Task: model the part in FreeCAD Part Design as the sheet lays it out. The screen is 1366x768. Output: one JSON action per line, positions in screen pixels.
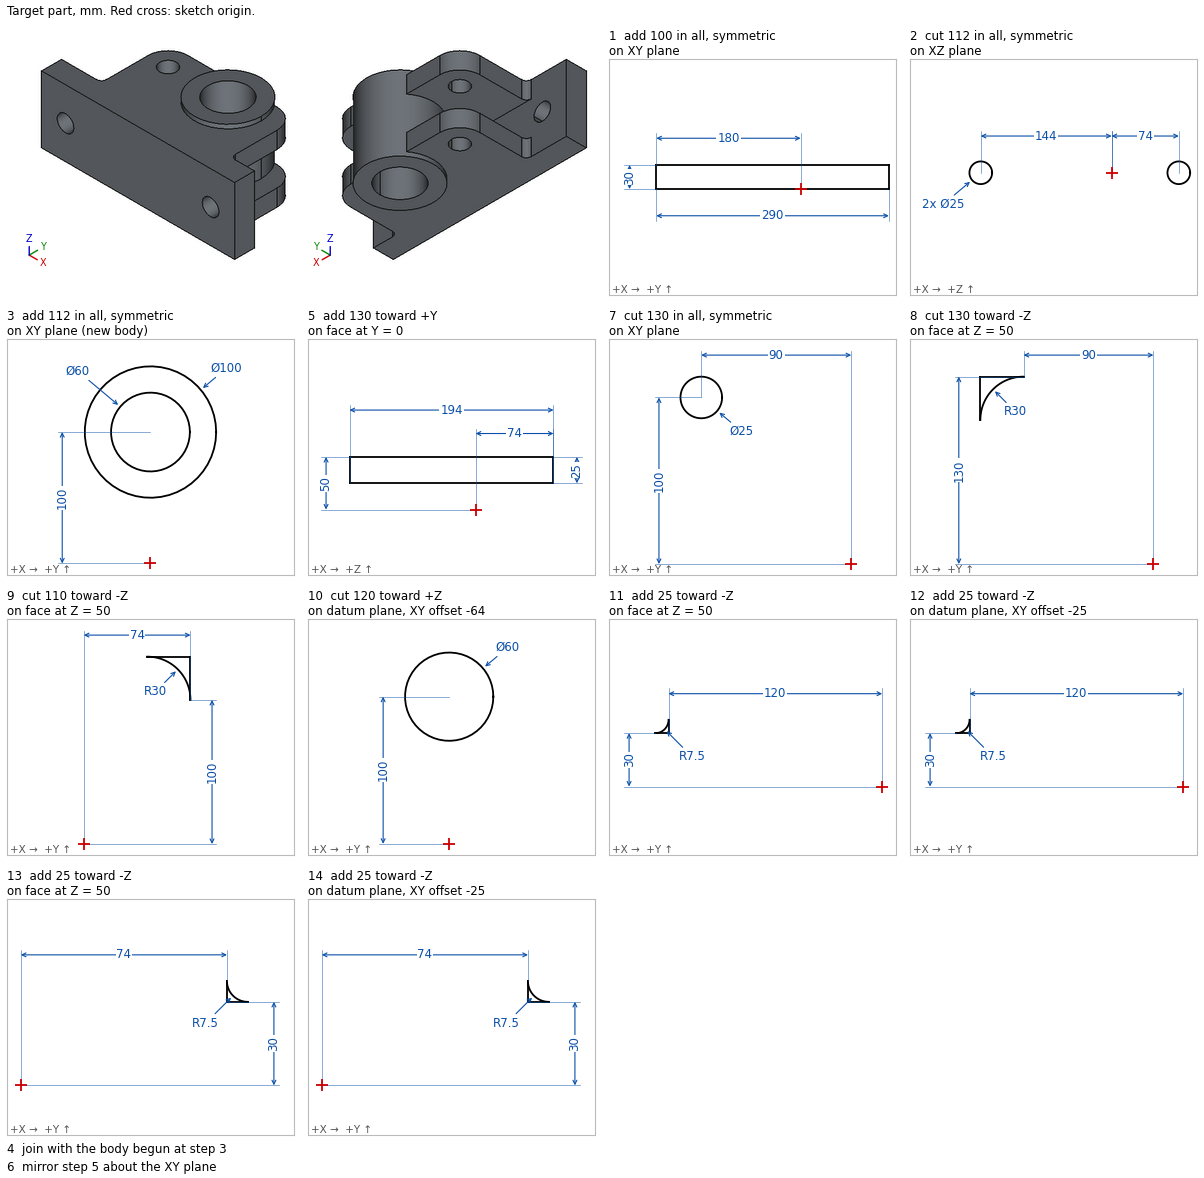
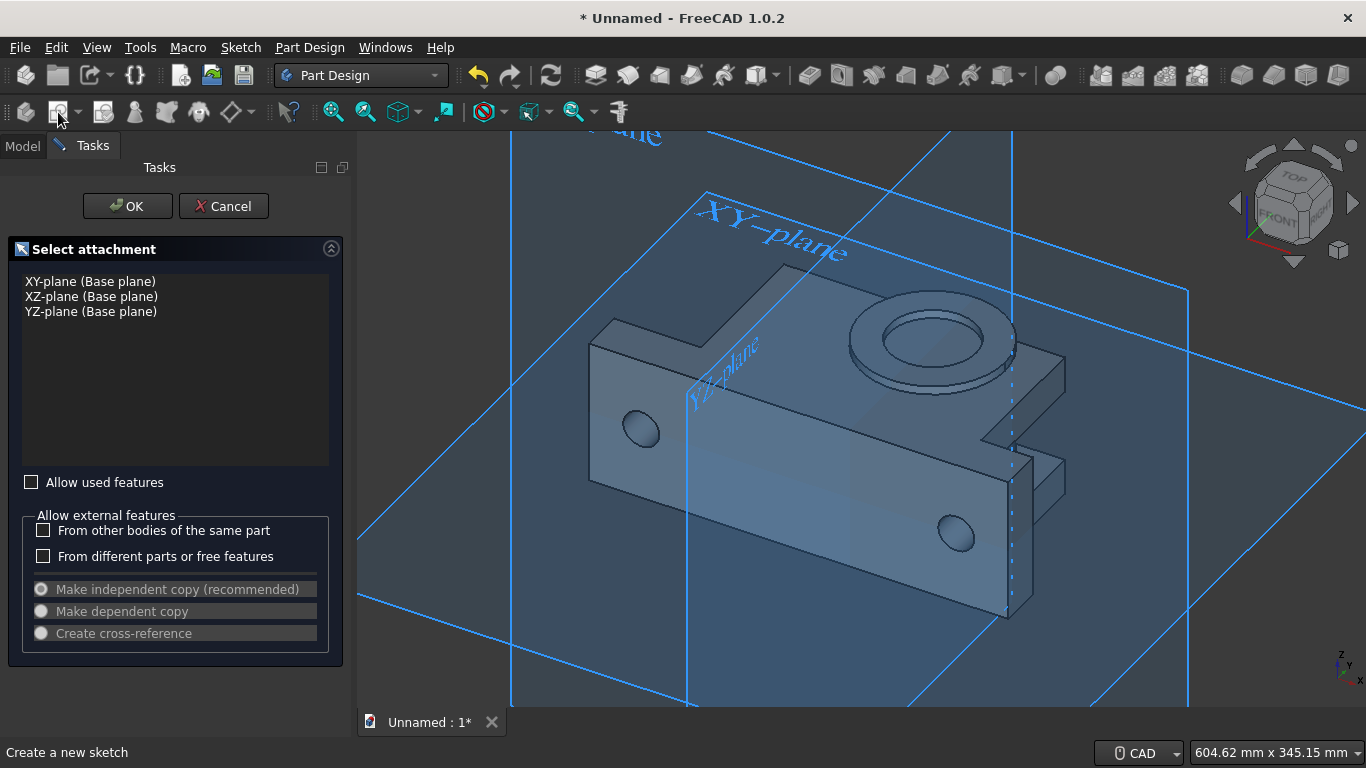
{"action": "left_click", "coordinate": [82, 282]}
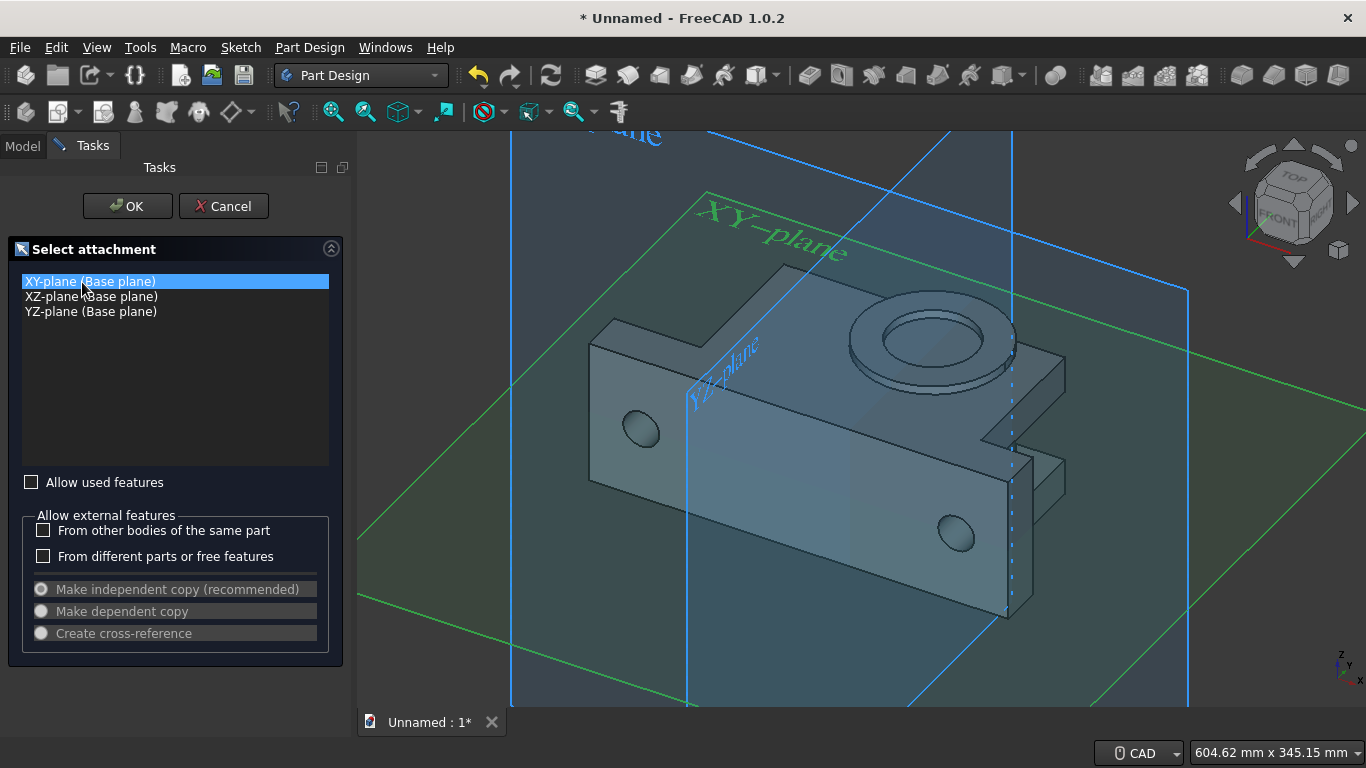
{"action": "left_click", "coordinate": [128, 206]}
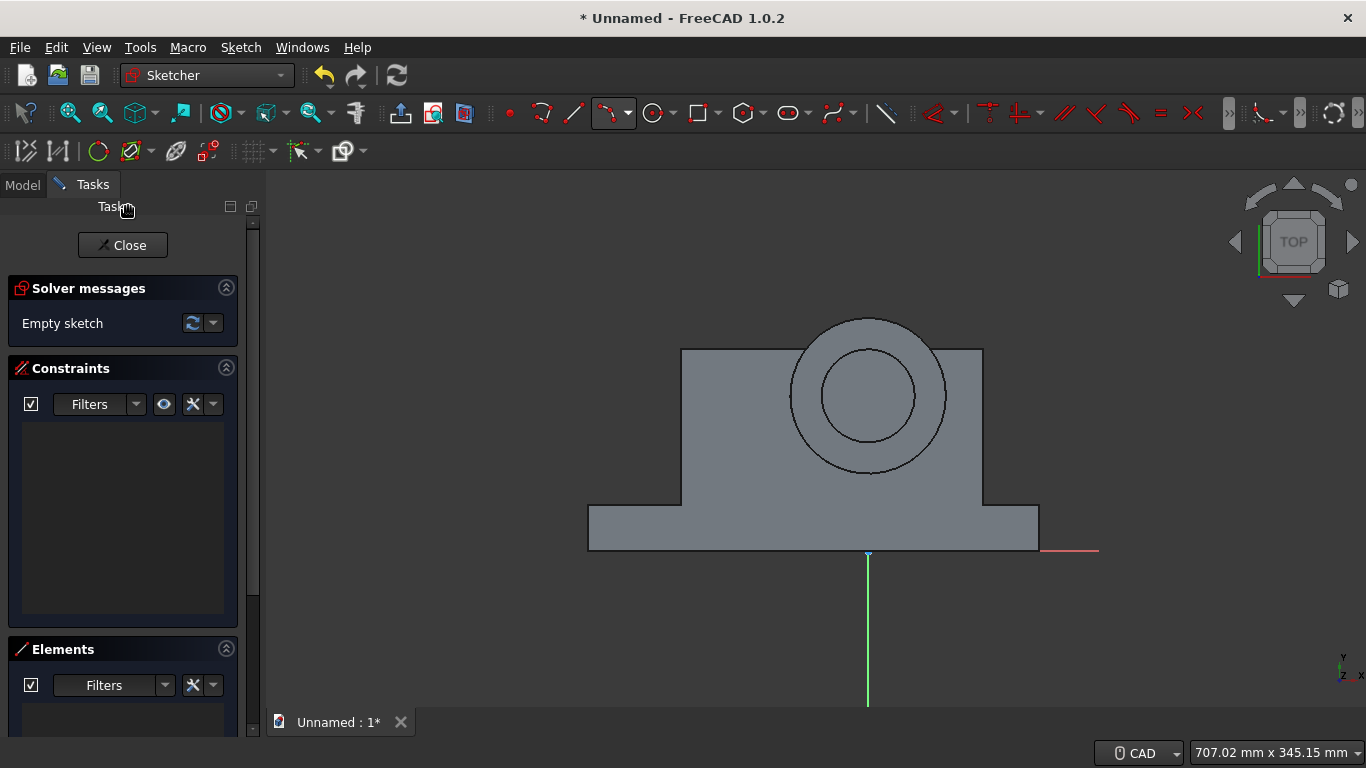
{"action": "left_click", "coordinate": [466, 114]}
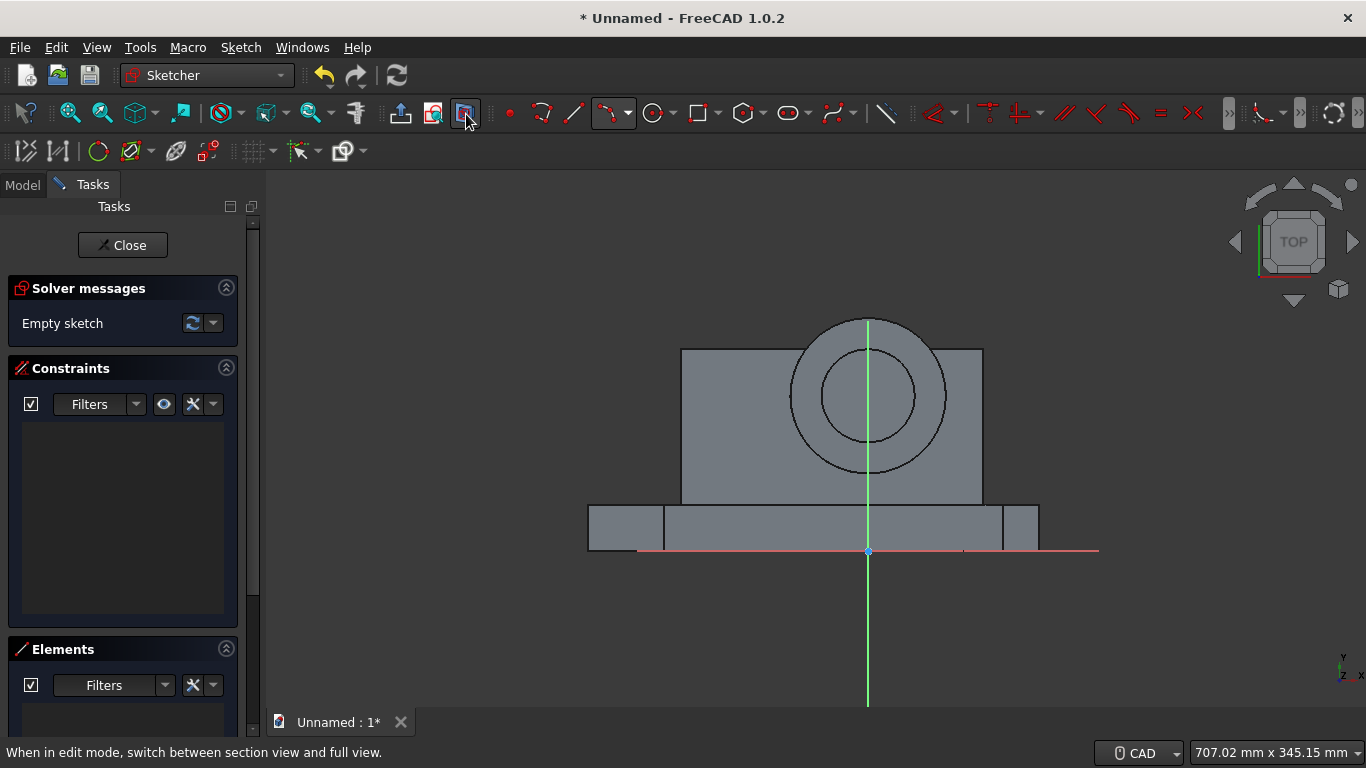
{"action": "scroll", "coordinate": [726, 391], "scroll_direction": "up", "scroll_amount": 11}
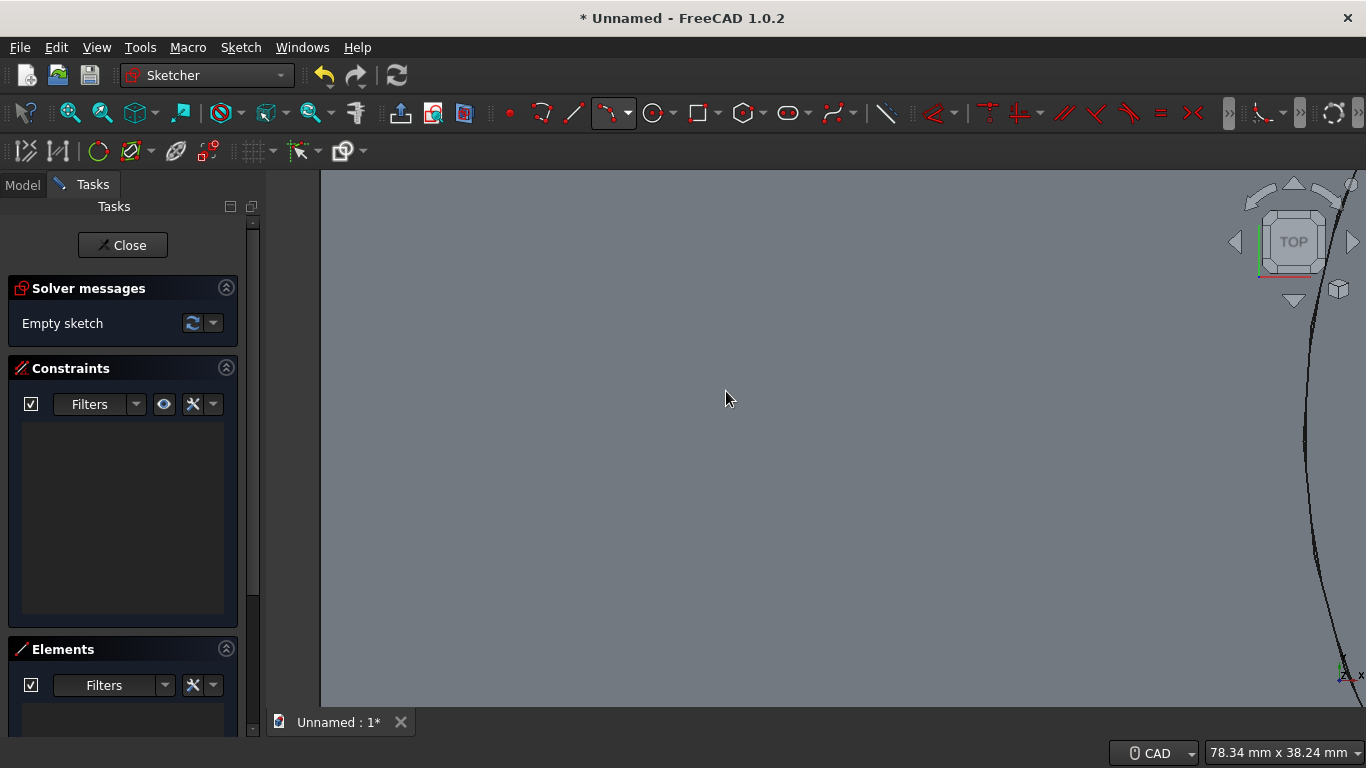
{"action": "left_click", "coordinate": [654, 114]}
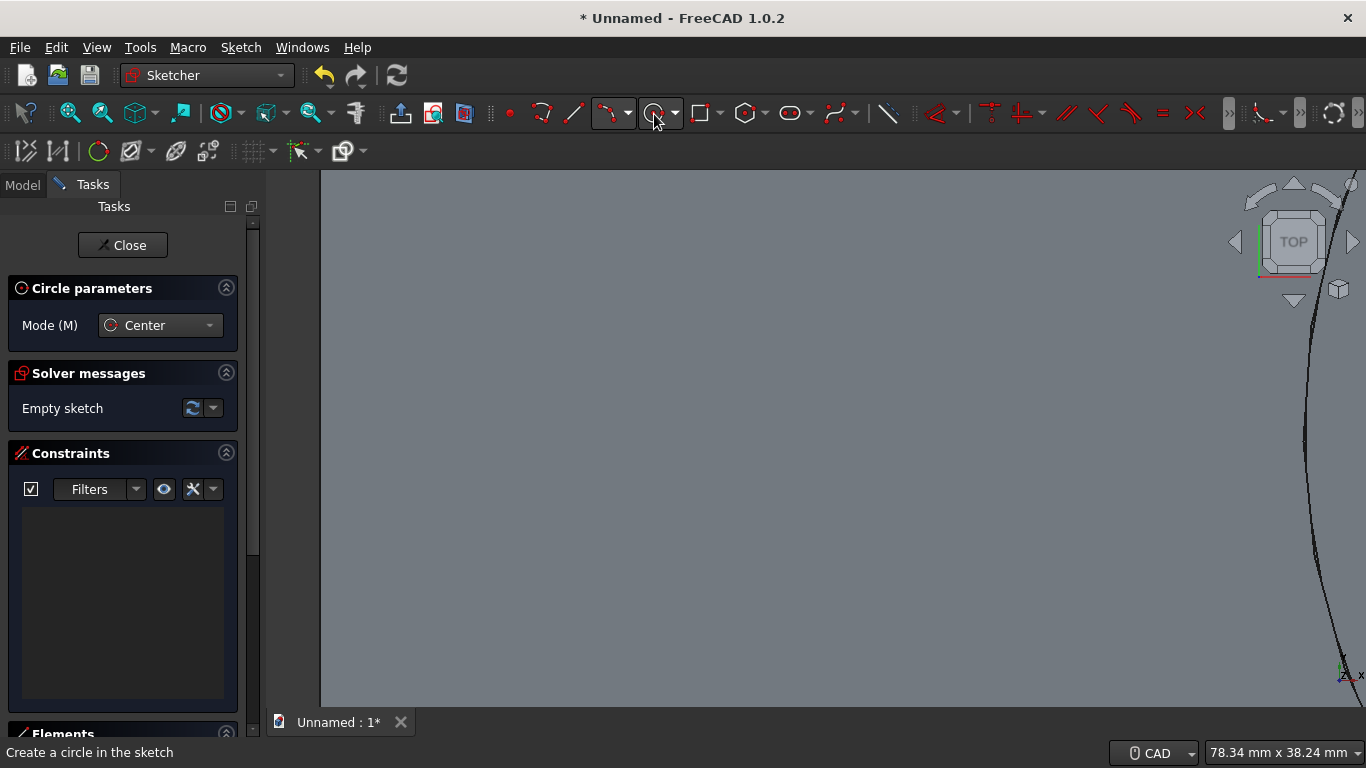
{"action": "left_click", "coordinate": [742, 431]}
{"action": "mouse_move", "coordinate": [866, 307]}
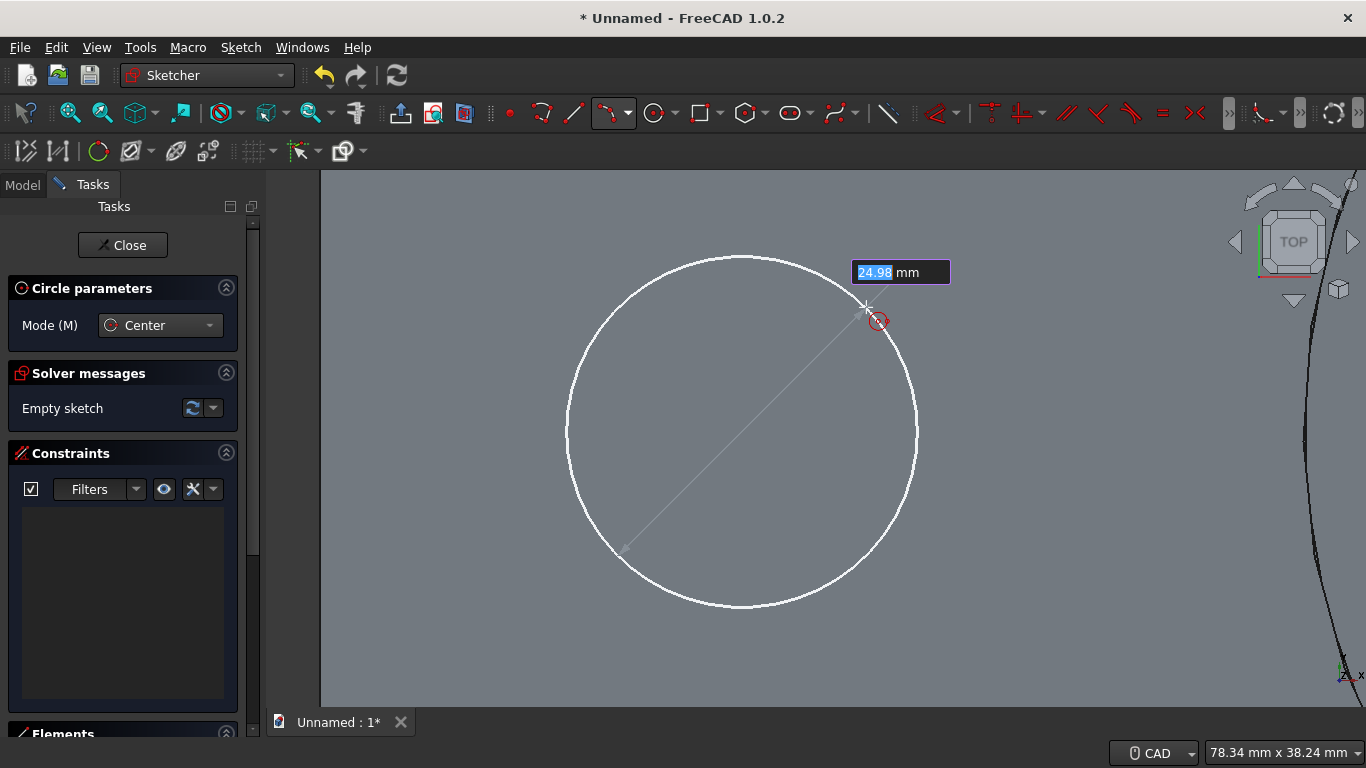
{"action": "type", "text": "25"}
{"action": "key", "text": "Return"}
{"action": "key", "text": "Escape"}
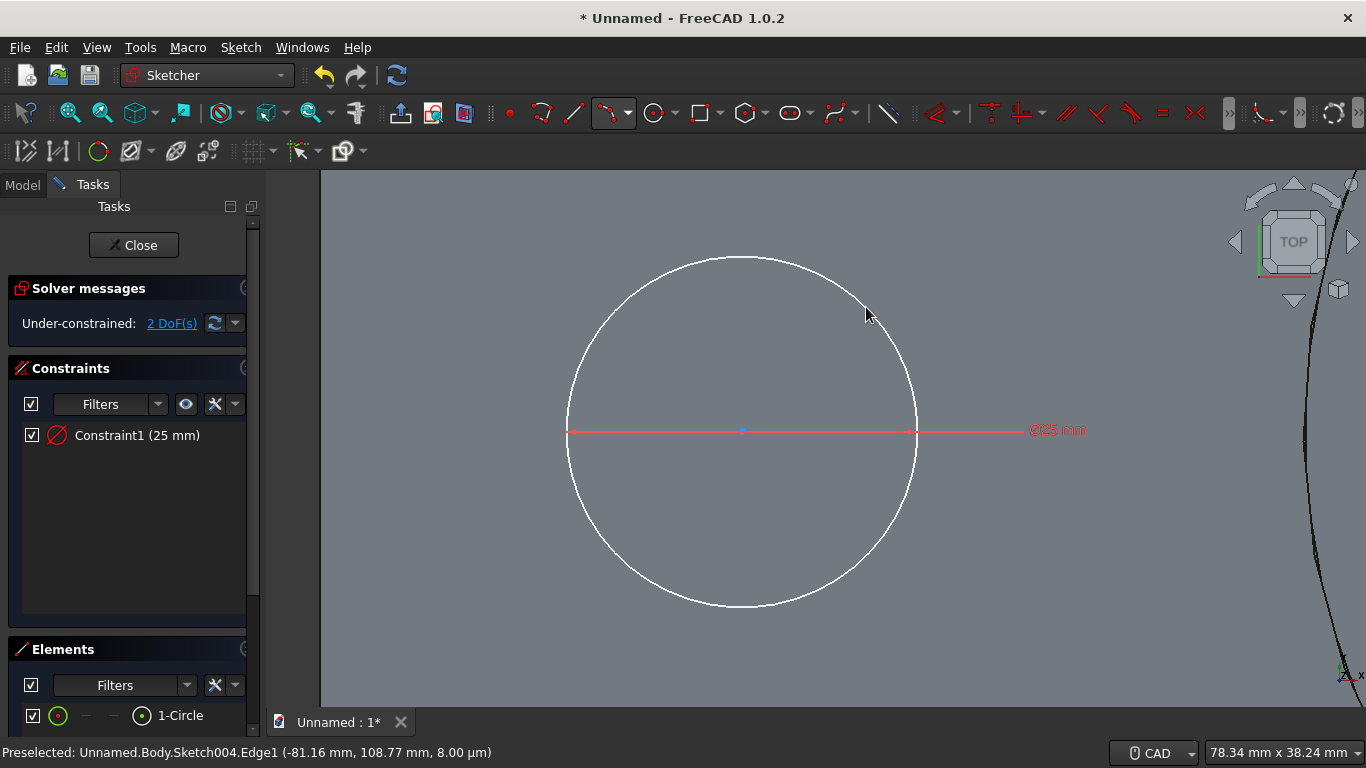
{"action": "left_click", "coordinate": [936, 114]}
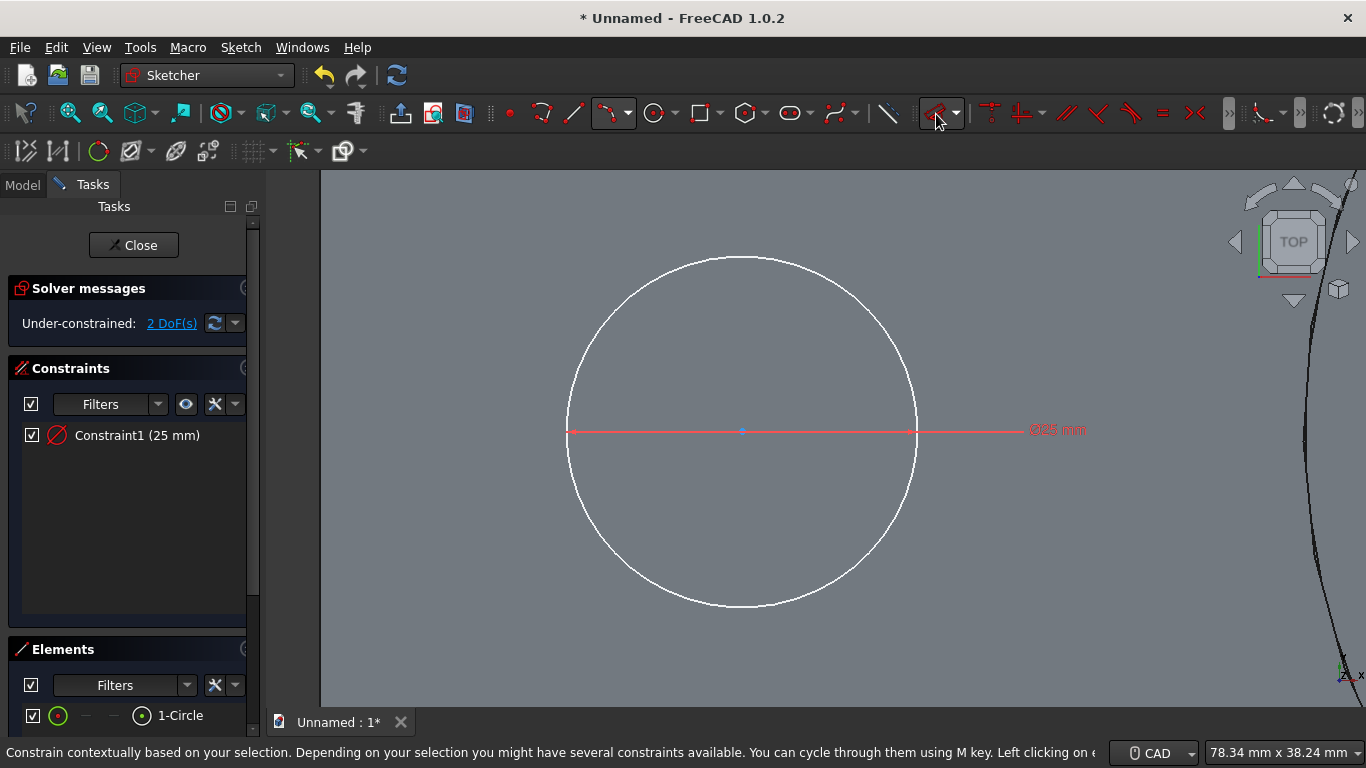
{"action": "left_click", "coordinate": [742, 432]}
{"action": "left_click", "coordinate": [972, 398]}